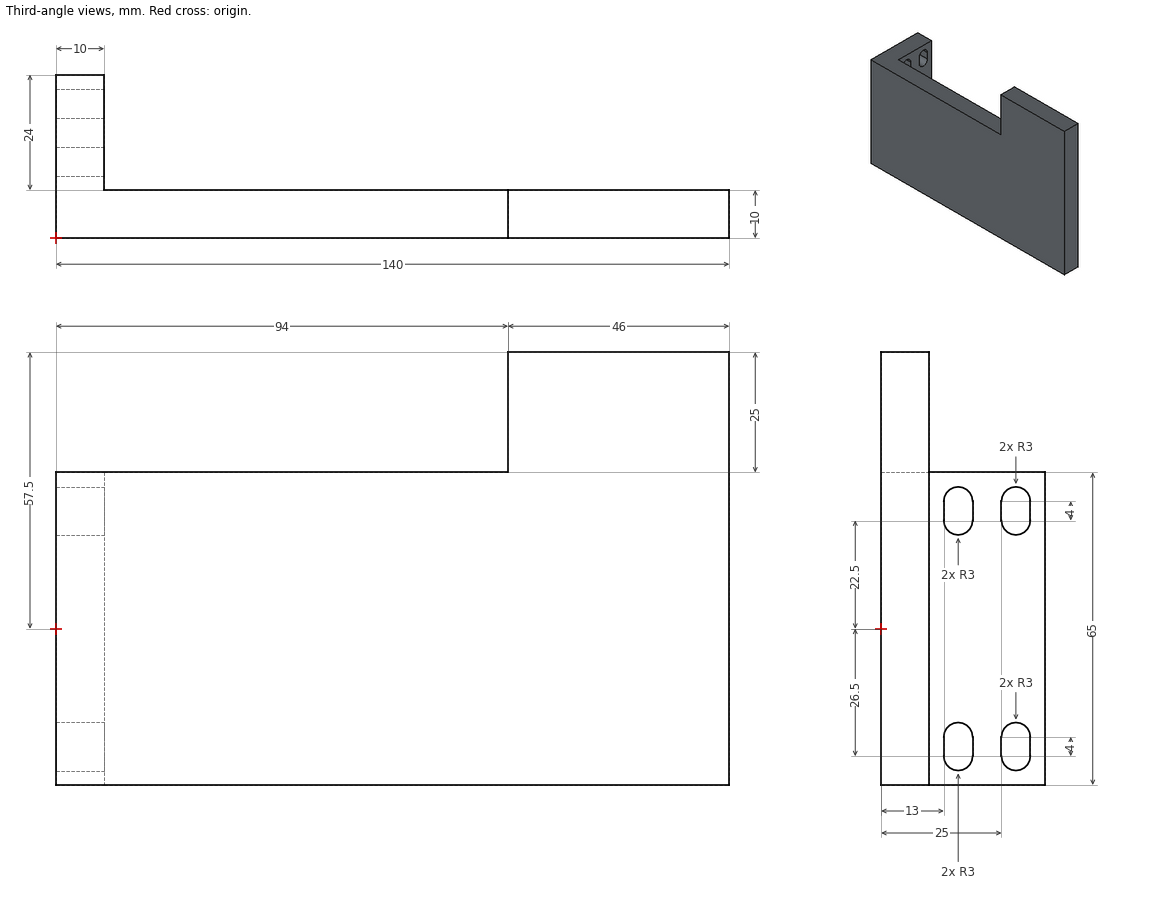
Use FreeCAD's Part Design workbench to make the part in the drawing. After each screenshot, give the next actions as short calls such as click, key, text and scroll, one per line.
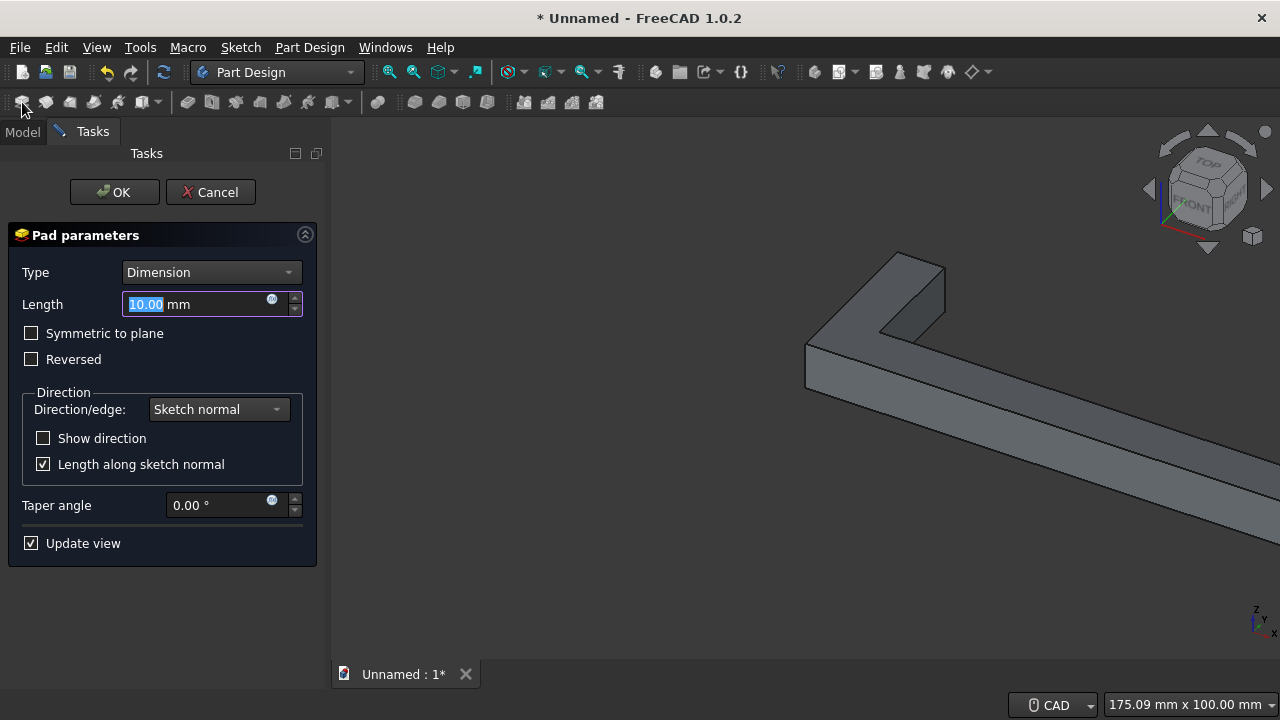
text(65)
key(Tab)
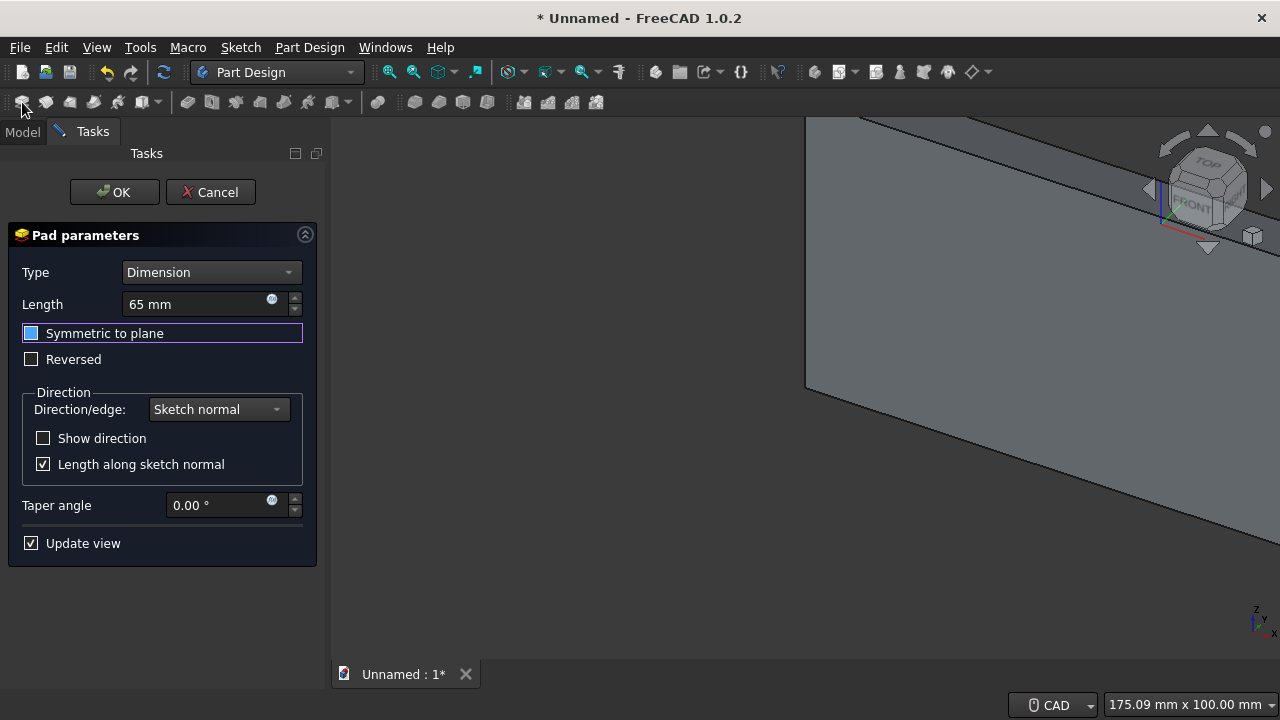
click(30, 333)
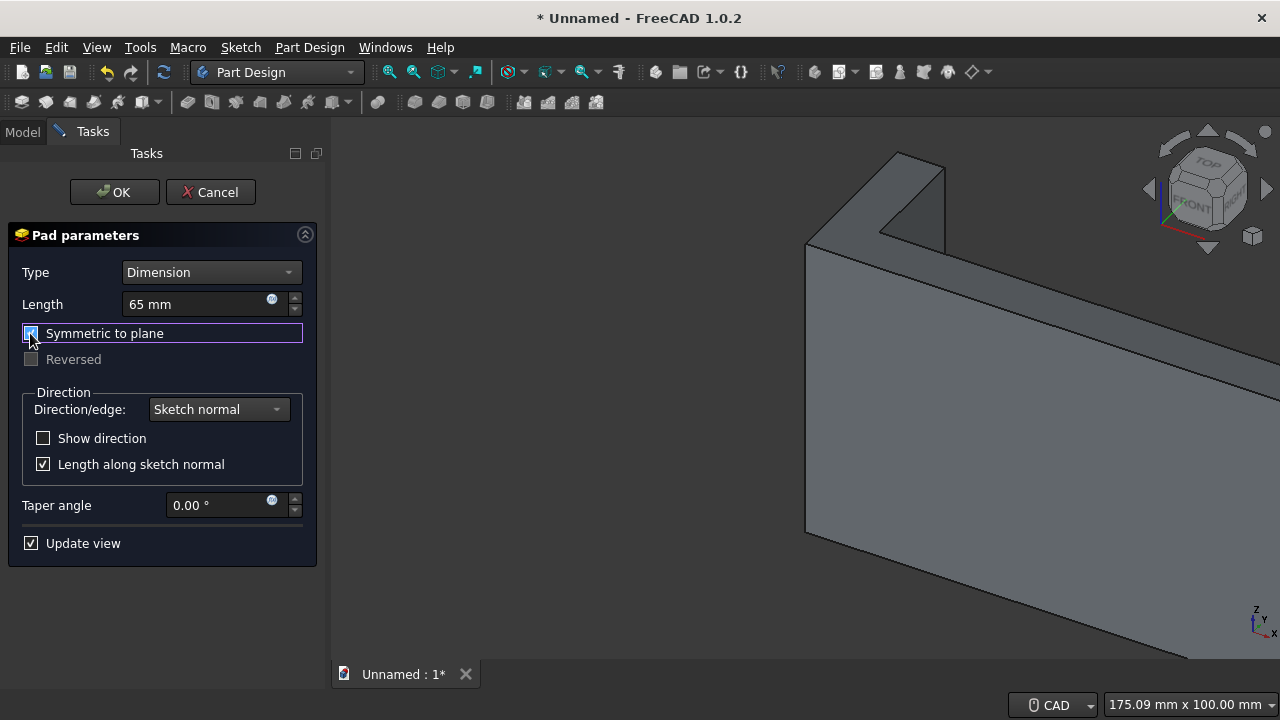
click(115, 192)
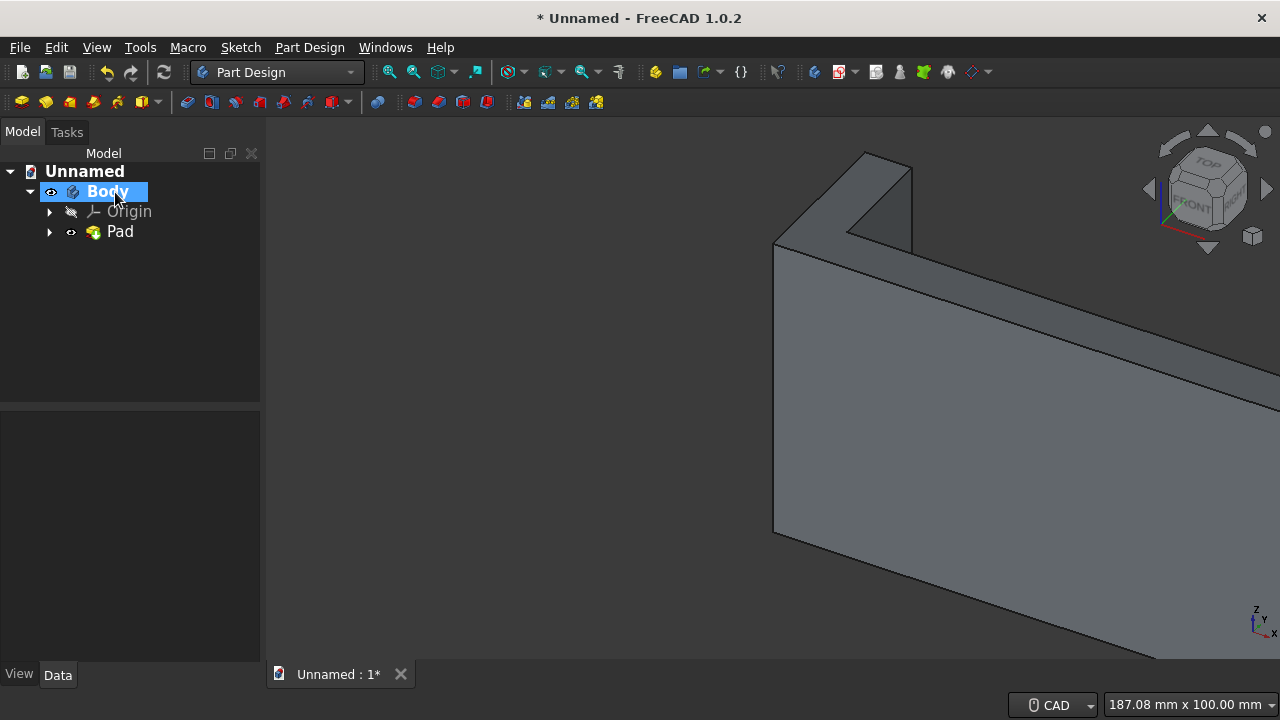
key(v)
key(f)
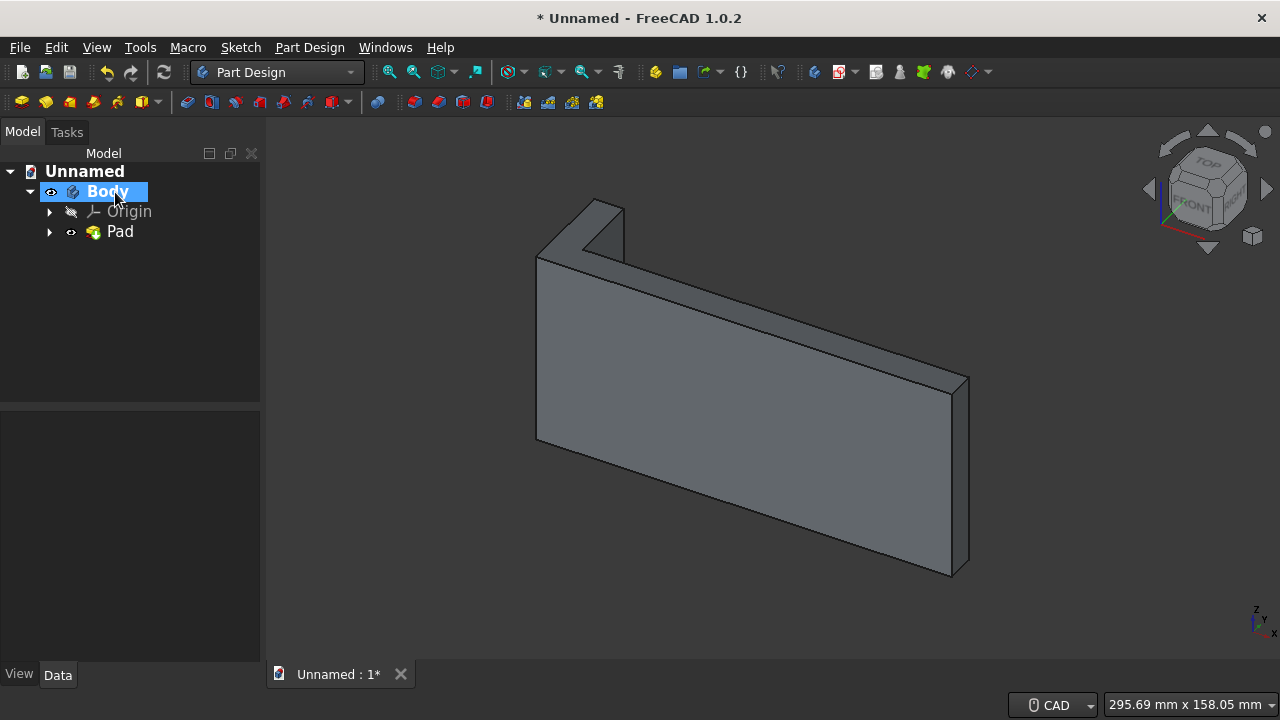
key(0)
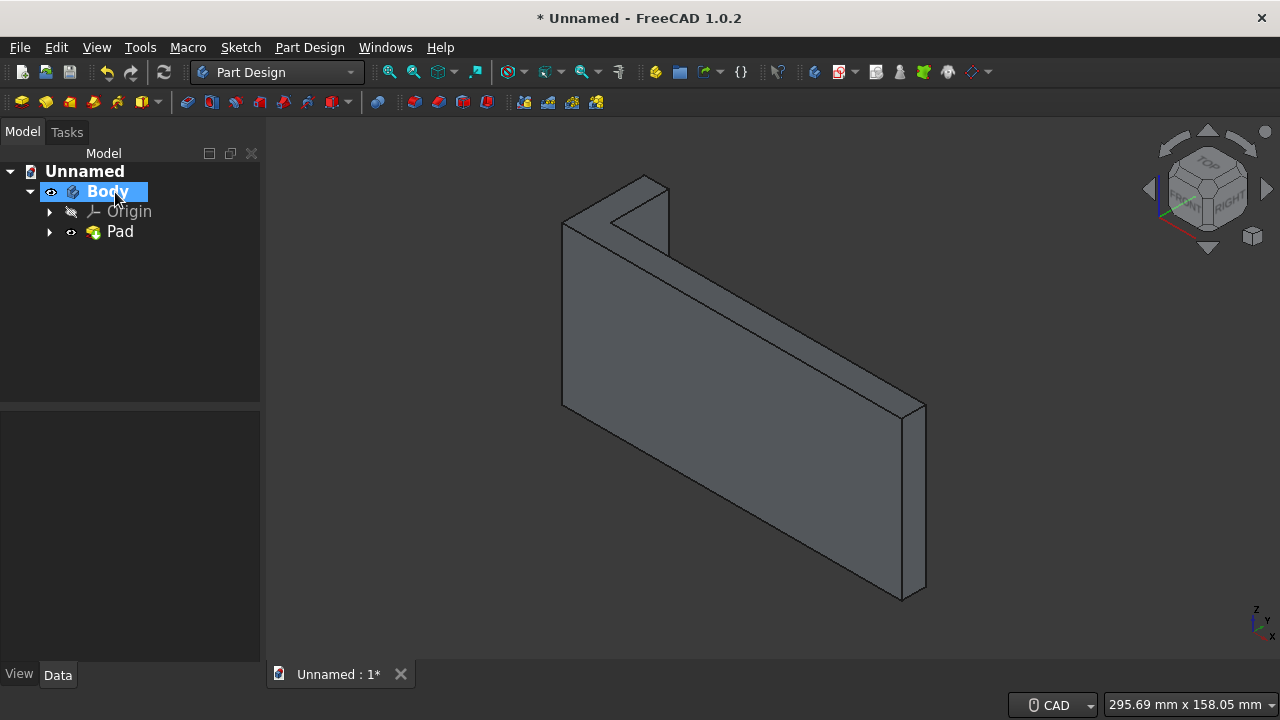
key(3)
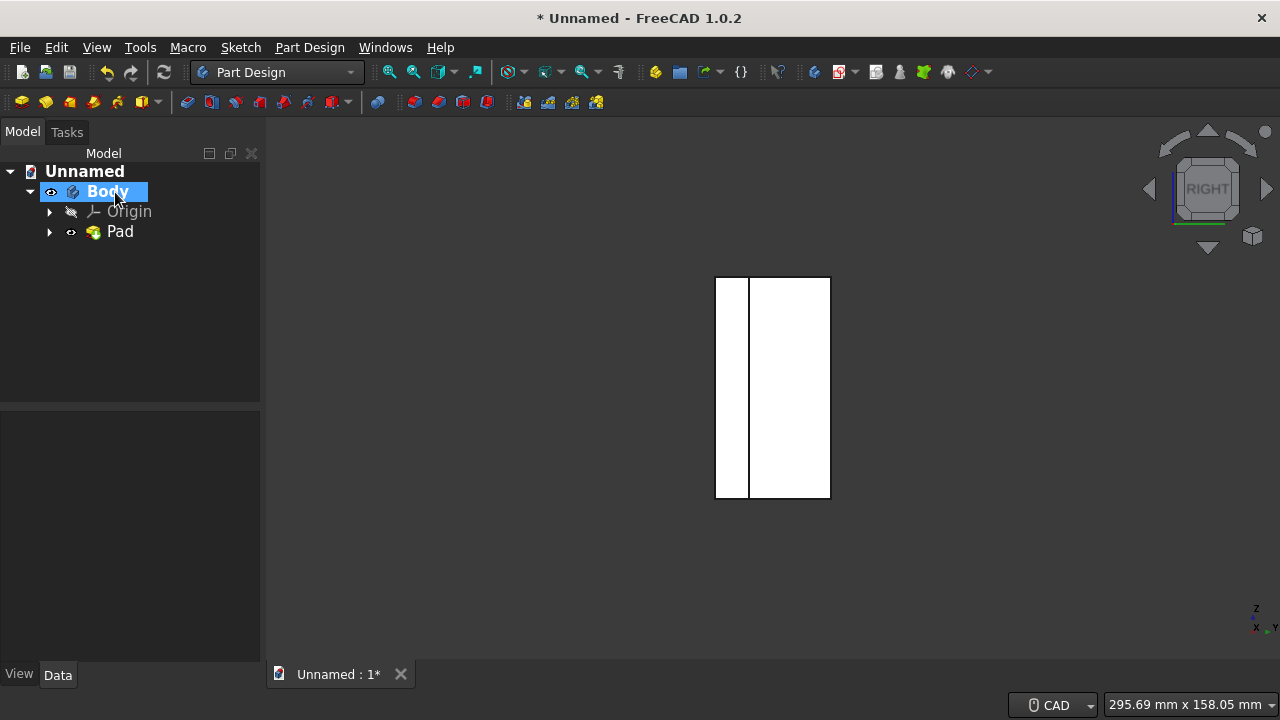
key(v)
key(f)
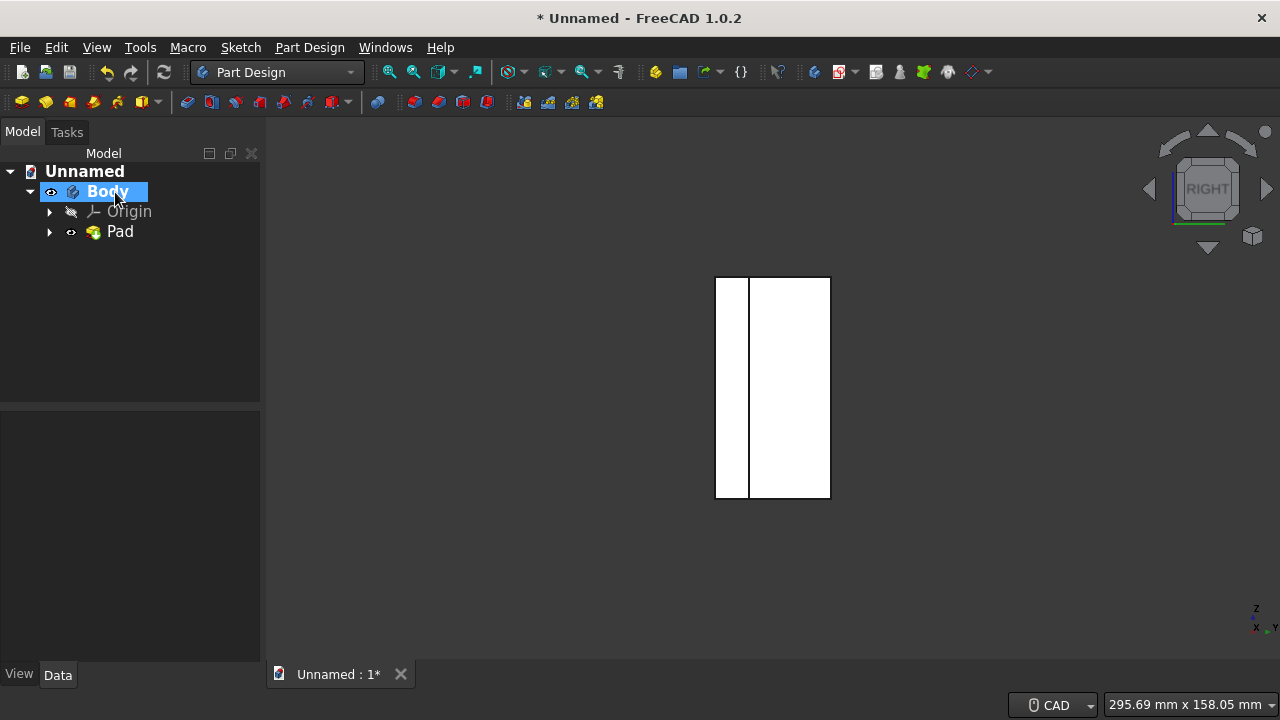
click(790, 323)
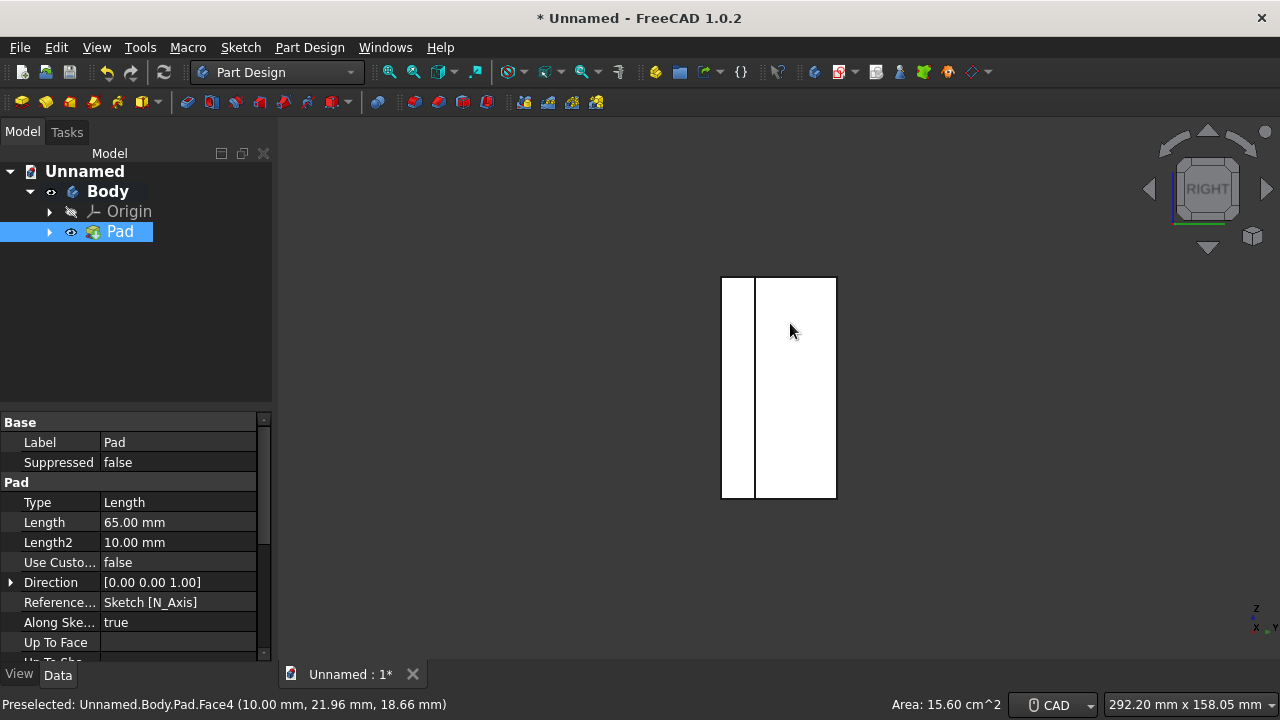
click(840, 72)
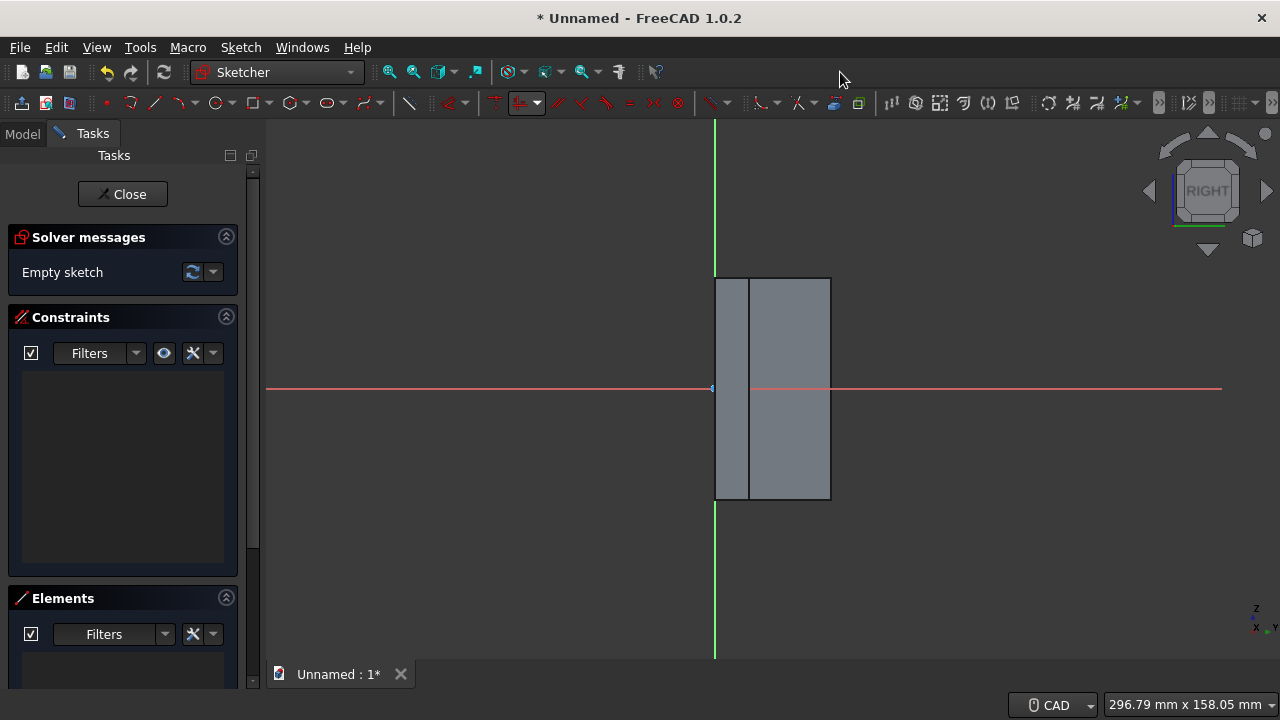
key(q)
key(s)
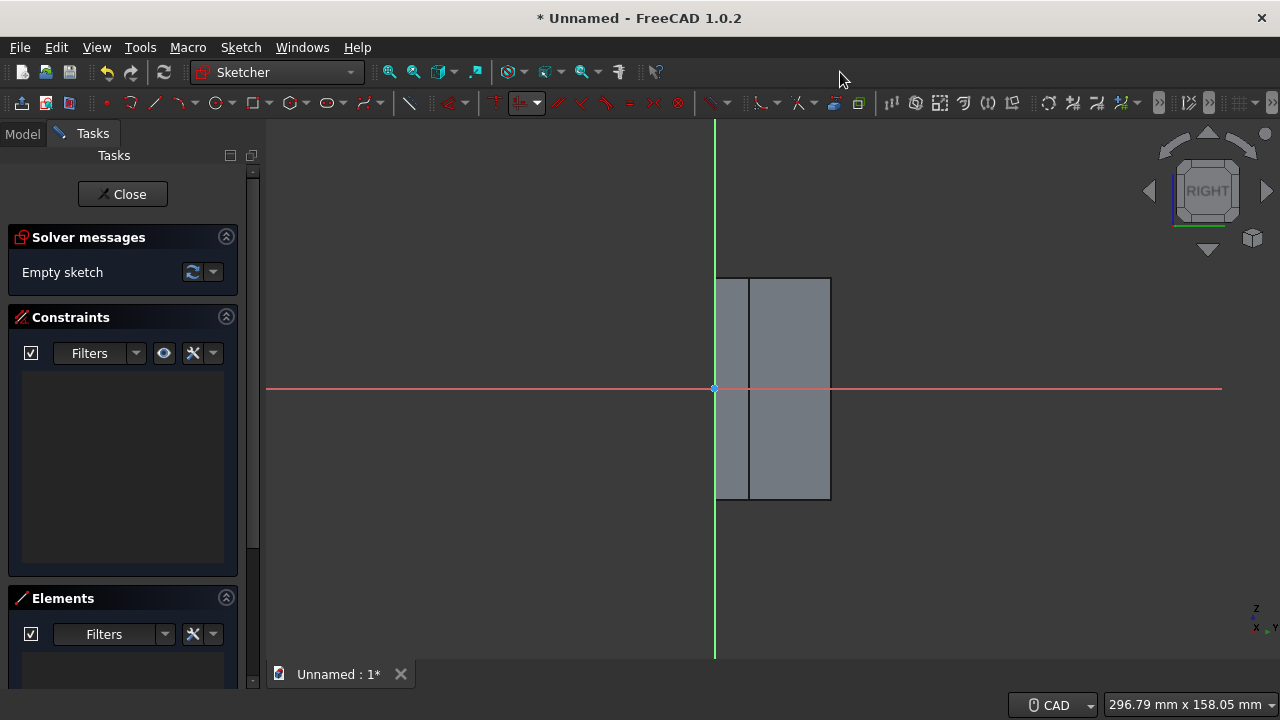
scroll(821, 297, up, 12)